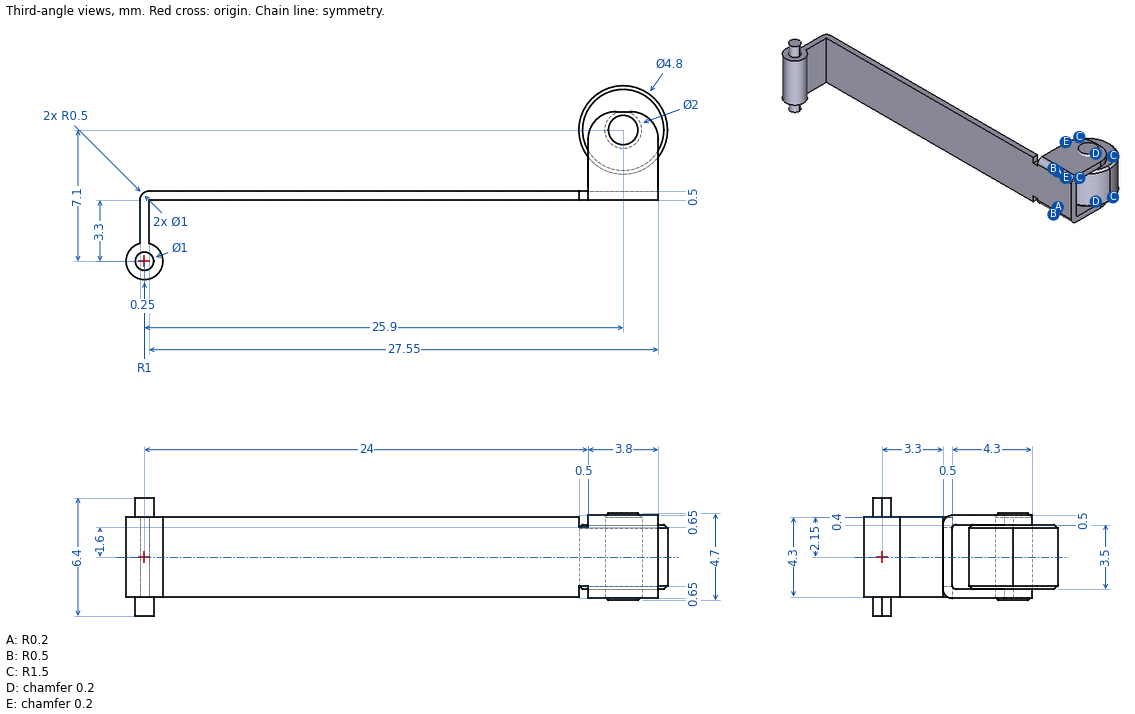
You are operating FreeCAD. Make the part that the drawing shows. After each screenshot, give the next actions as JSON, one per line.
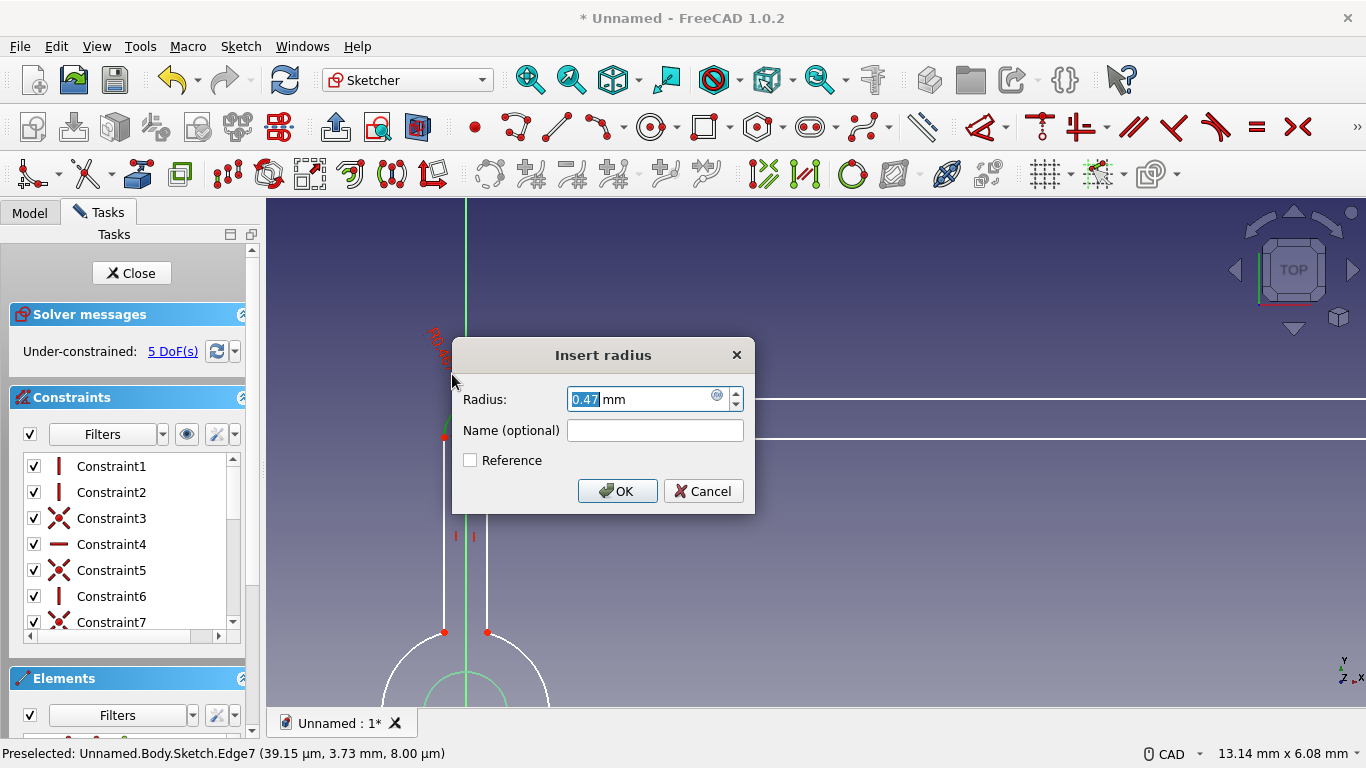
{"action": "type", "text": "0.5"}
{"action": "key", "text": "Return"}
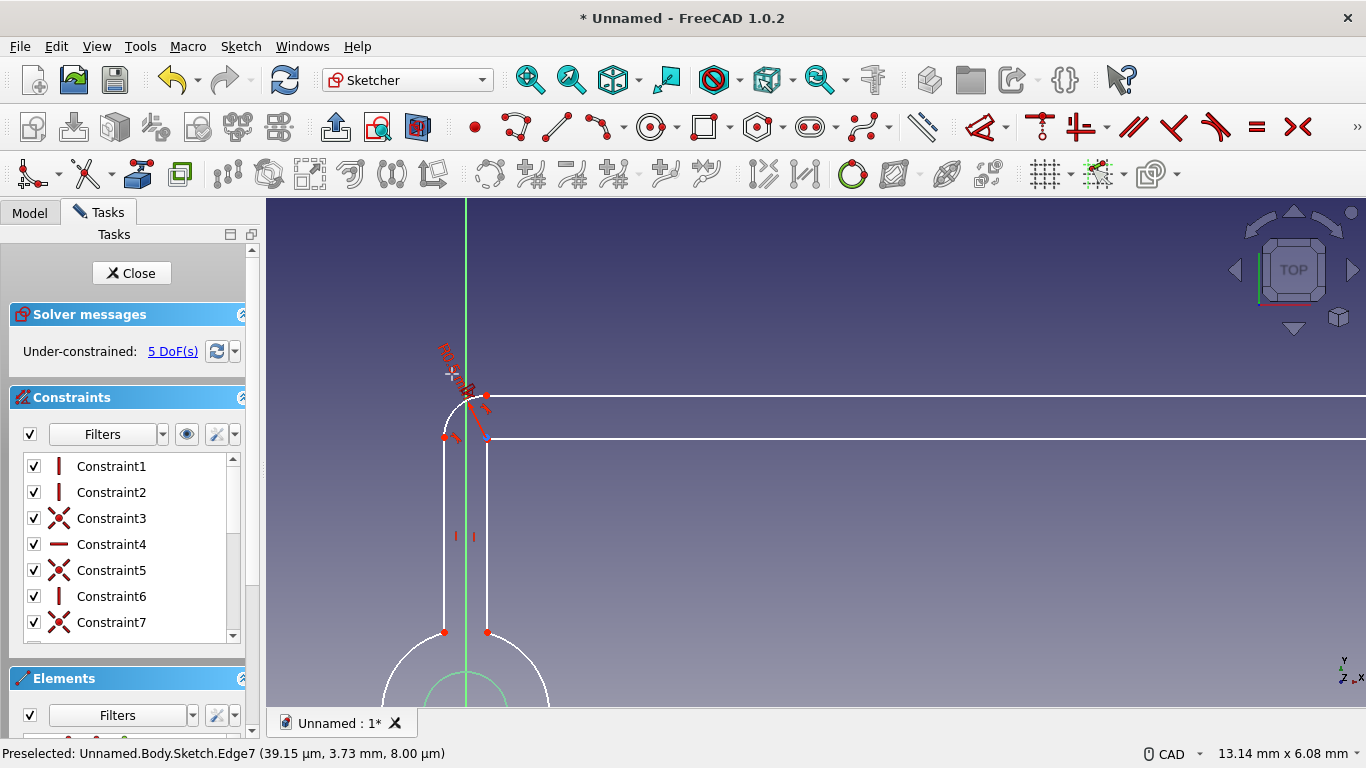
{"action": "scroll", "coordinate": [466, 405], "scroll_direction": "down", "scroll_amount": 7}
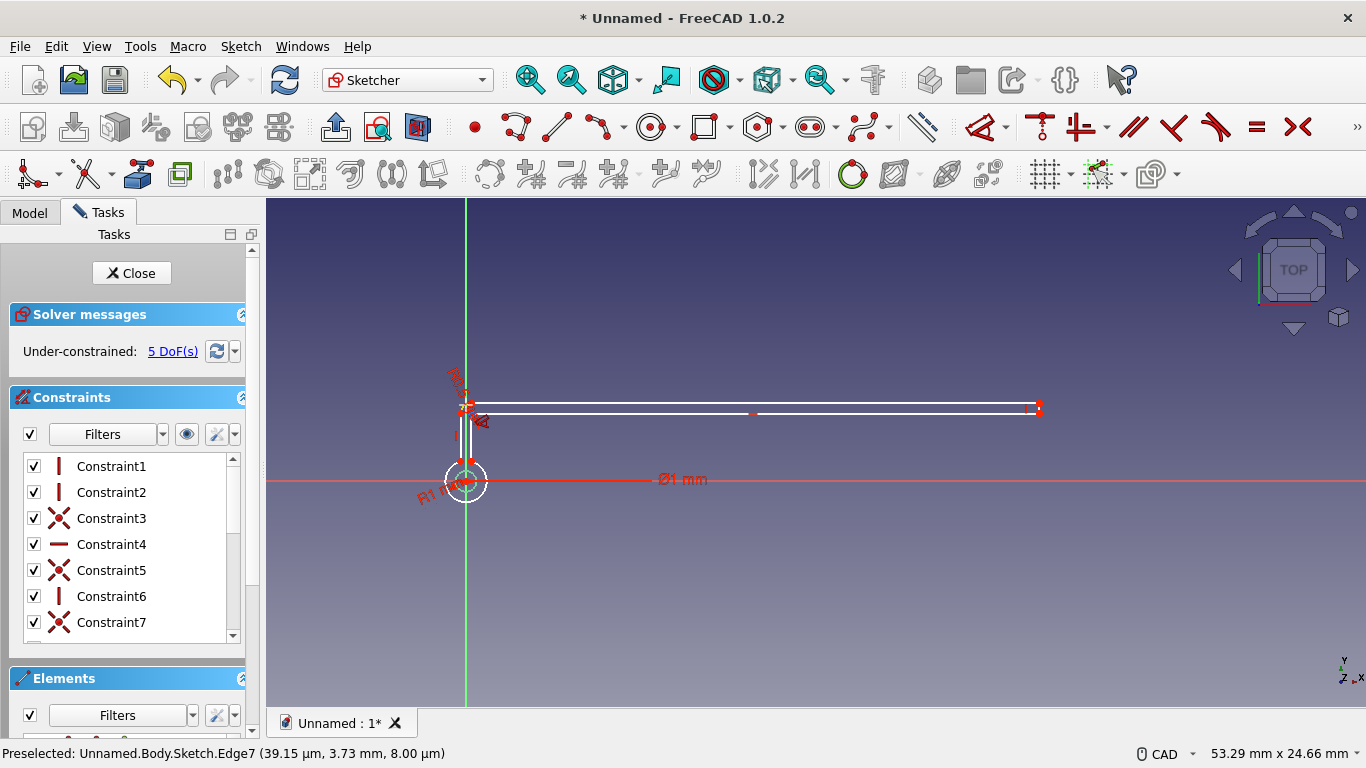
{"action": "scroll", "coordinate": [1039, 411], "scroll_direction": "up", "scroll_amount": 8}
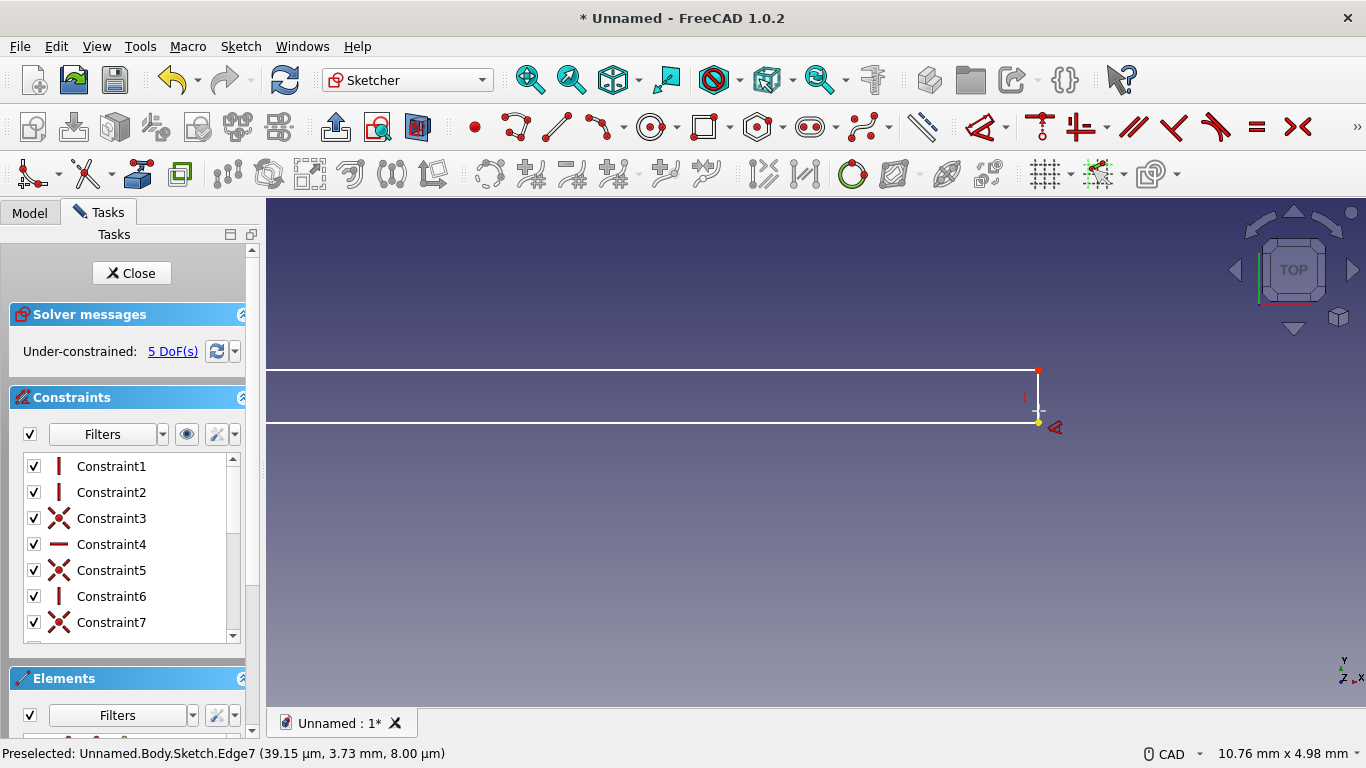
{"action": "left_click", "coordinate": [1038, 407]}
{"action": "left_click", "coordinate": [1072, 396]}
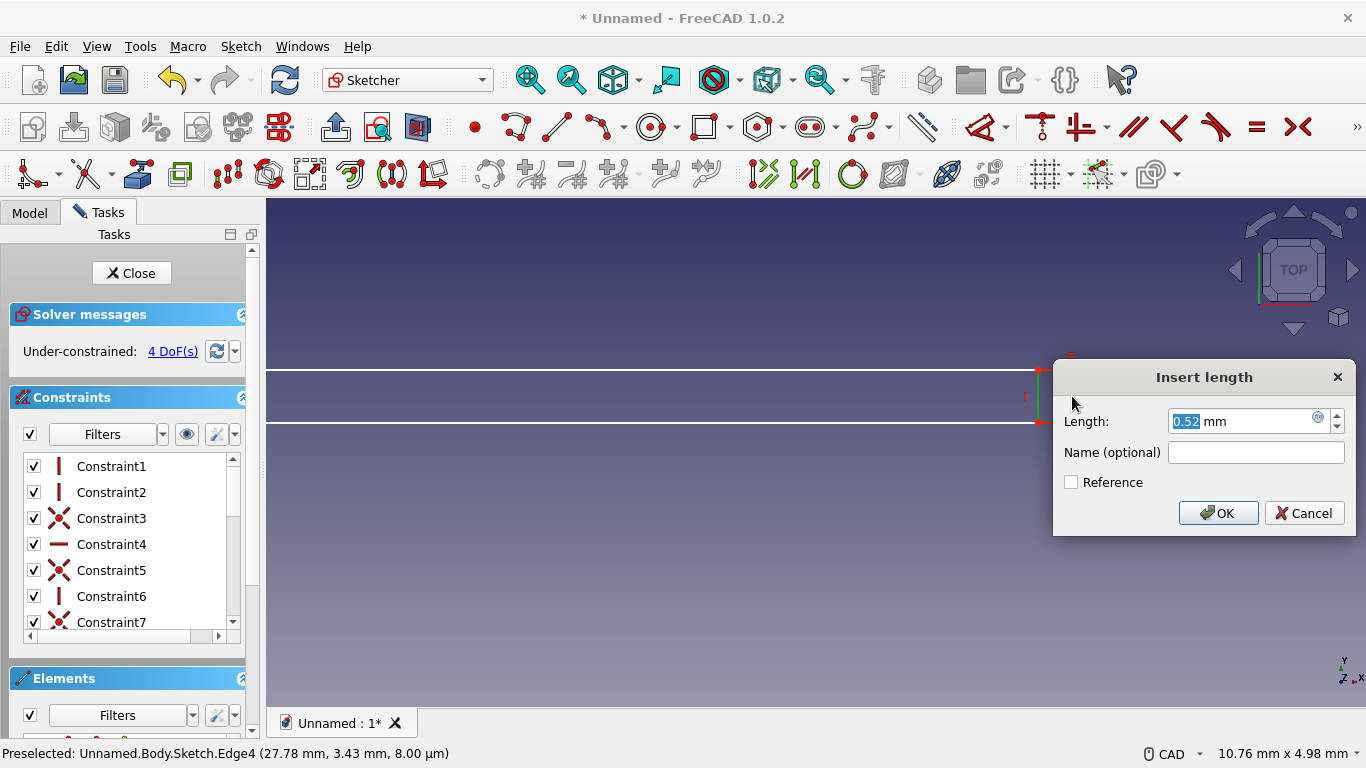
{"action": "type", "text": "0.5"}
{"action": "key", "text": "Return"}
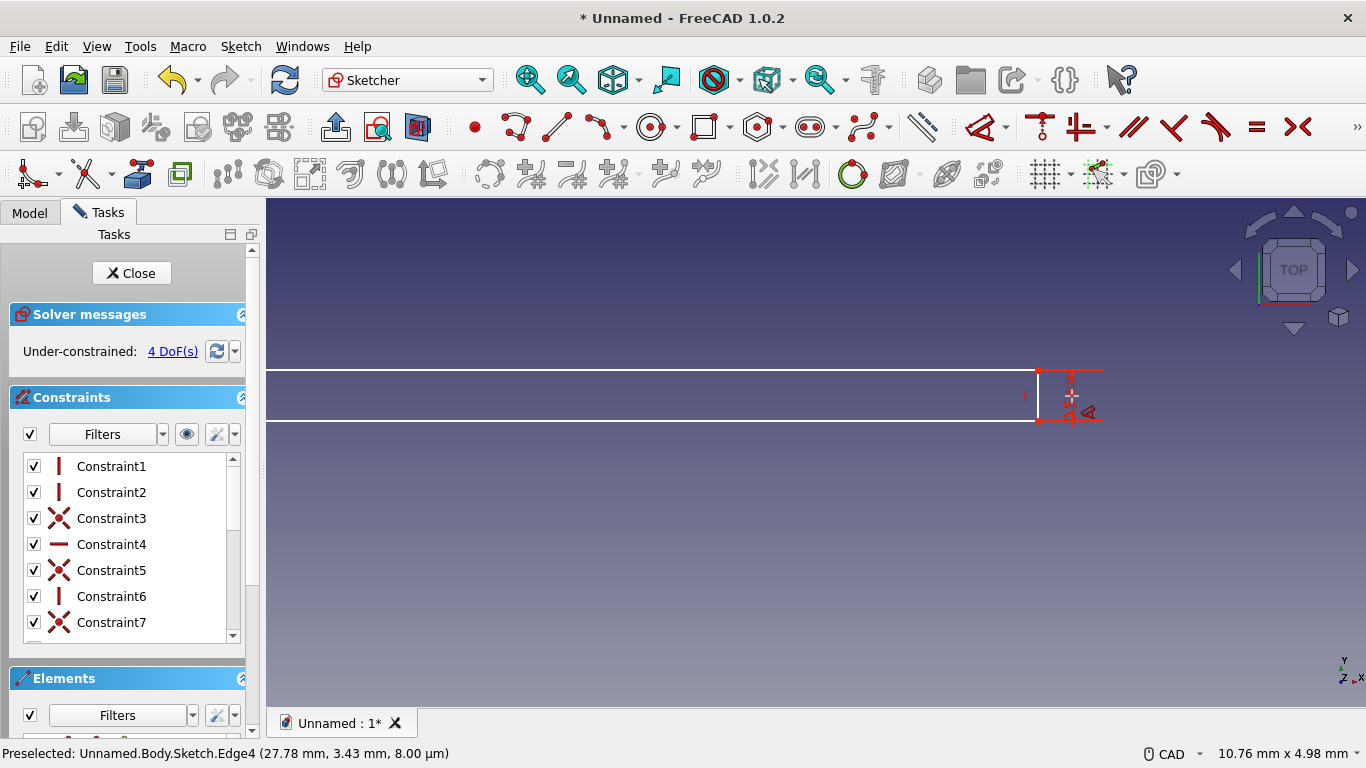
{"action": "scroll", "coordinate": [1039, 411], "scroll_direction": "down", "scroll_amount": 8}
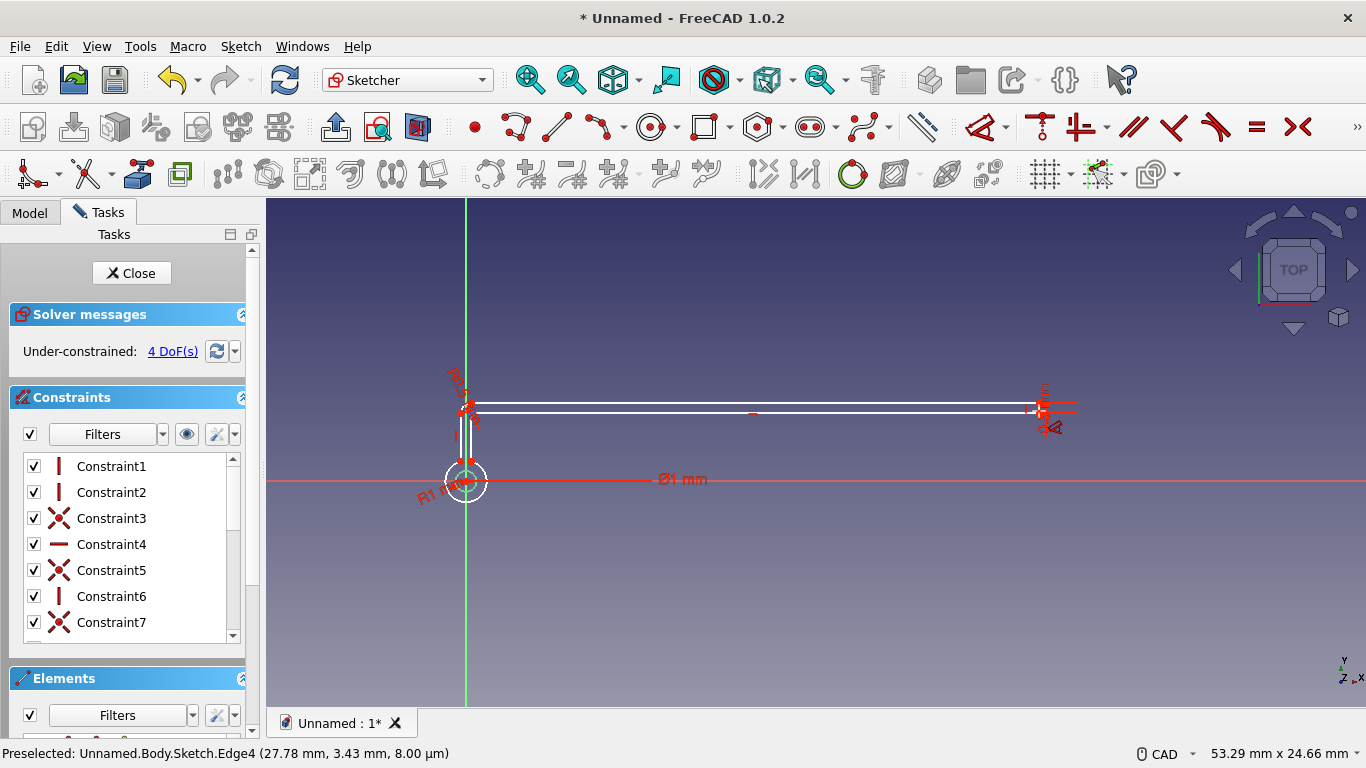
{"action": "left_click", "coordinate": [461, 413]}
{"action": "left_click", "coordinate": [427, 447]}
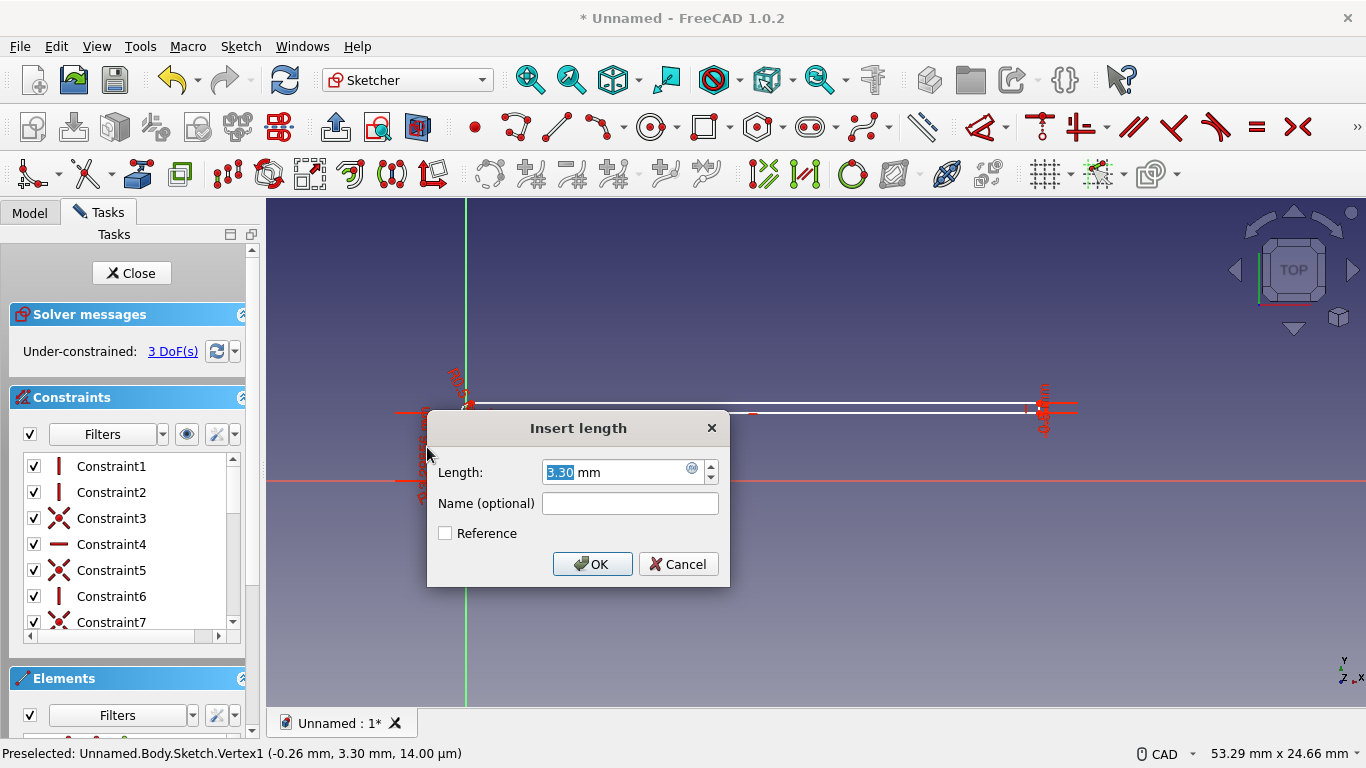
{"action": "type", "text": "3.3"}
{"action": "key", "text": "Return"}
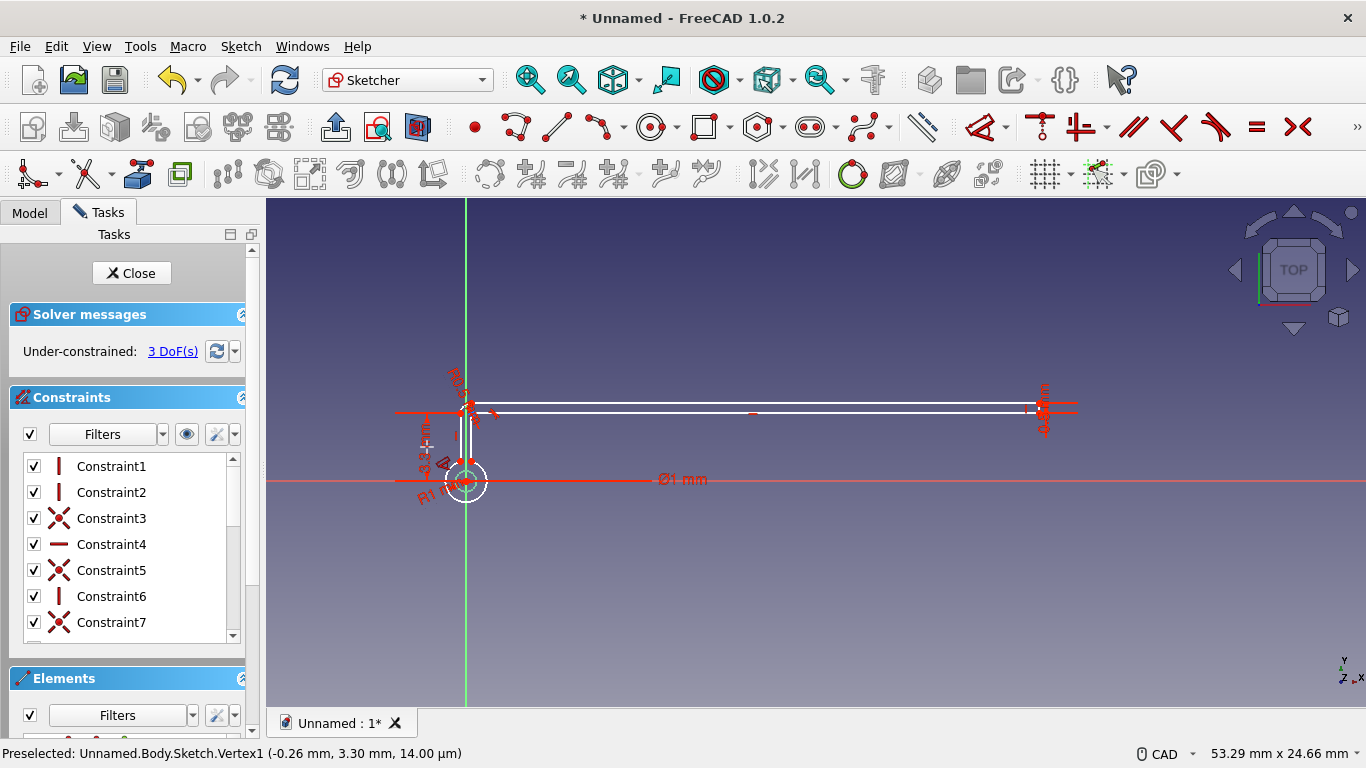
{"action": "scroll", "coordinate": [642, 413], "scroll_direction": "up", "scroll_amount": 2}